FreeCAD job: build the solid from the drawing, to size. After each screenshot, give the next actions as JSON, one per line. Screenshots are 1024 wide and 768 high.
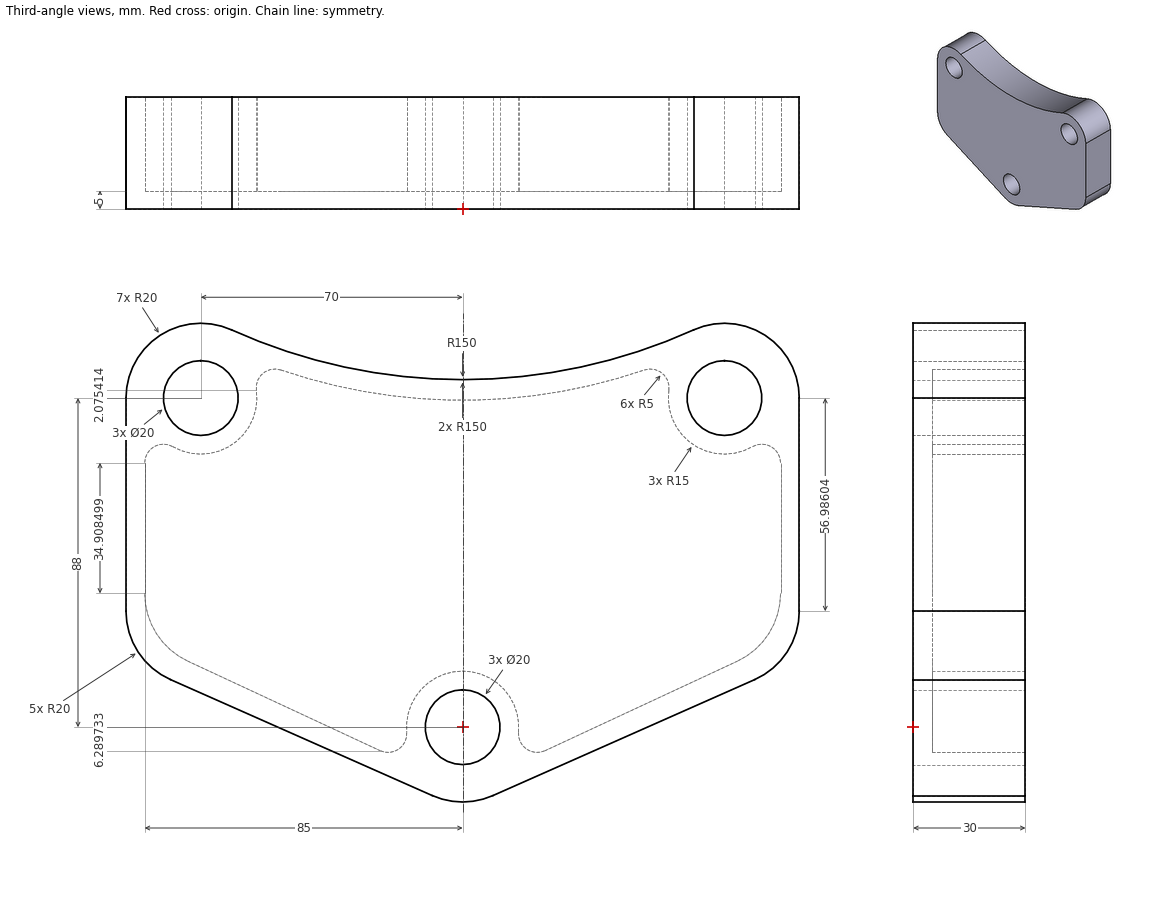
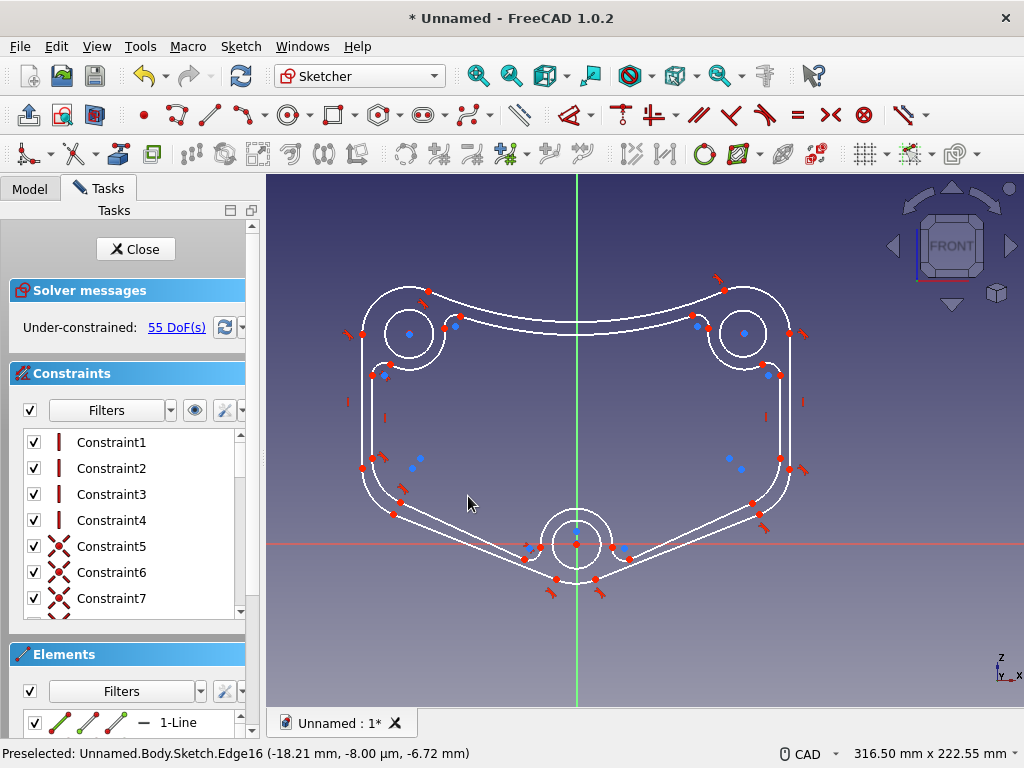
{"action": "scroll", "coordinate": [666, 543], "scroll_direction": "up", "scroll_amount": 3}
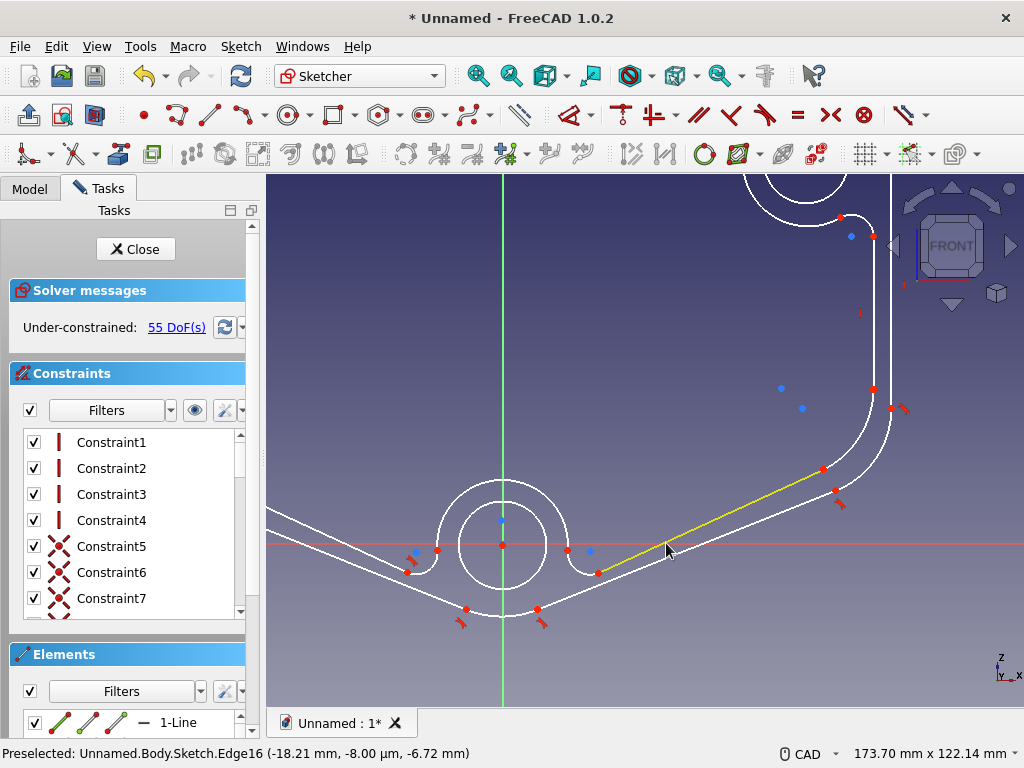
{"action": "left_click", "coordinate": [666, 542]}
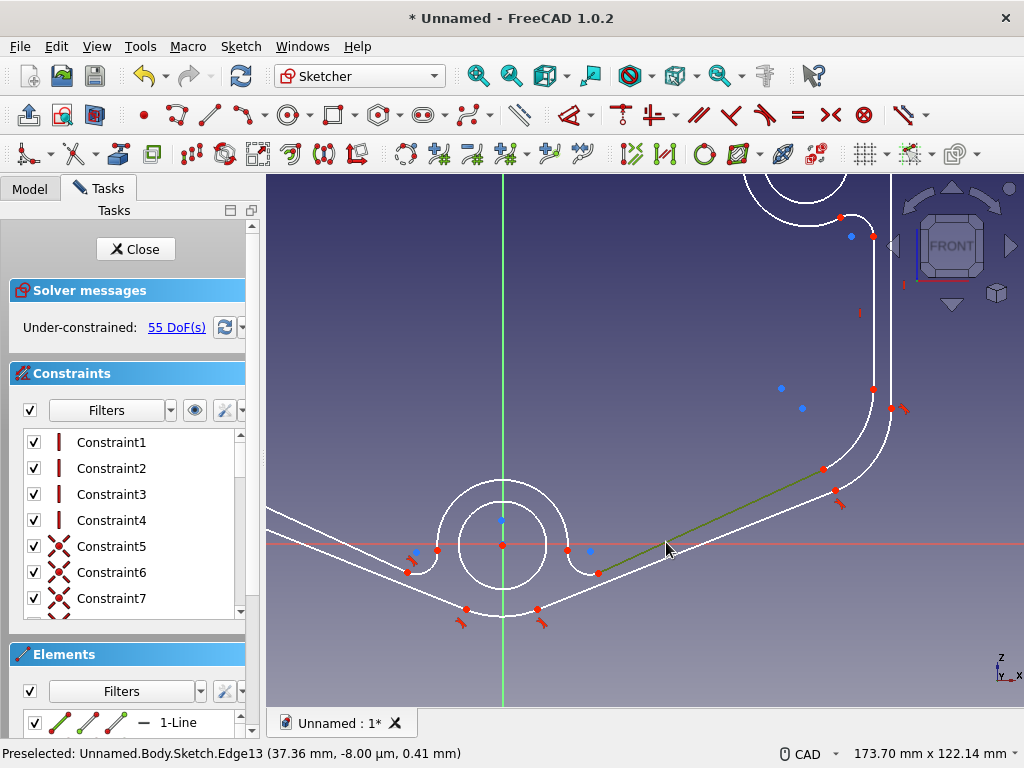
{"action": "left_click", "coordinate": [571, 563]}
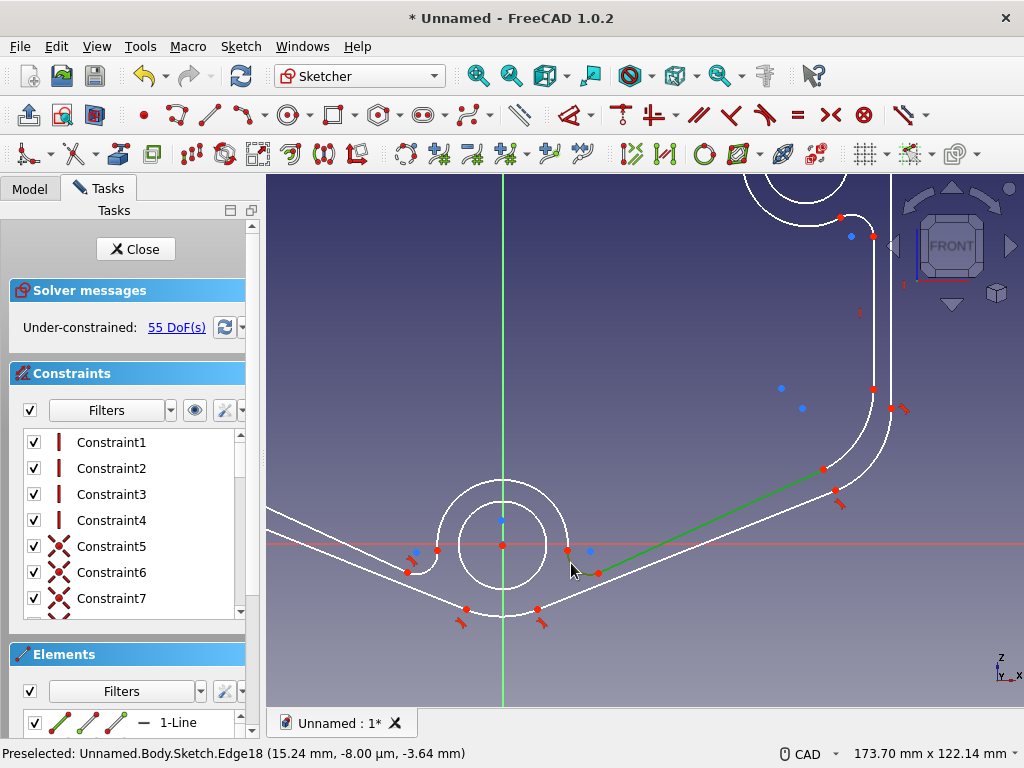
{"action": "left_click", "coordinate": [765, 116]}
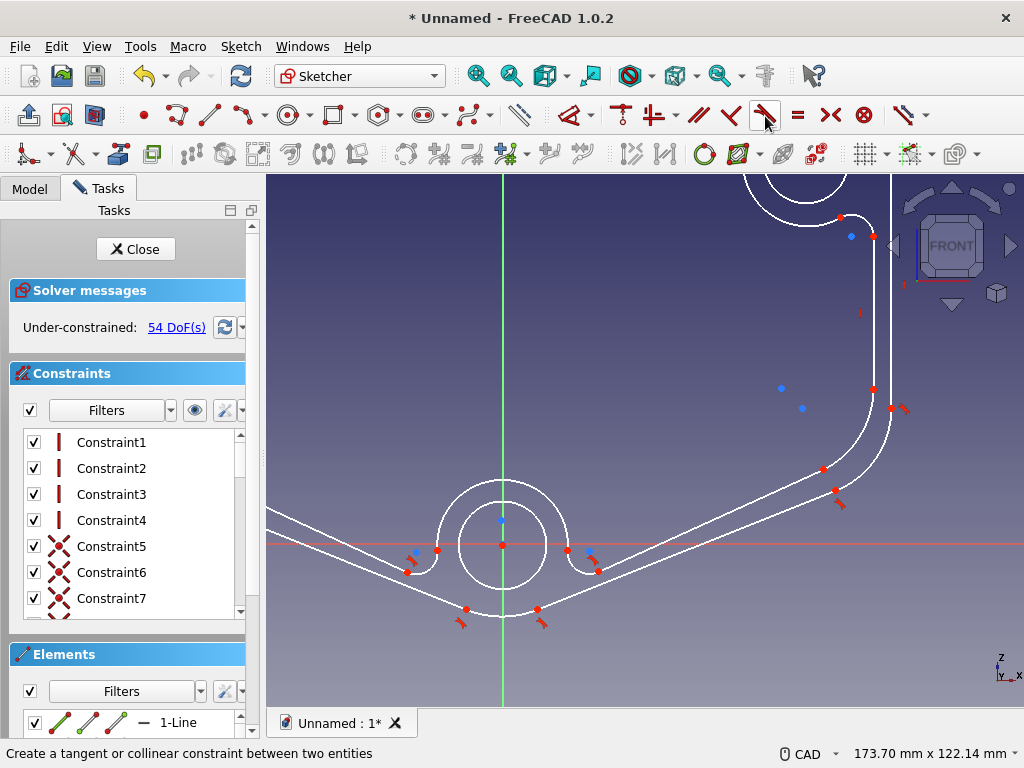
{"action": "left_click", "coordinate": [666, 541]}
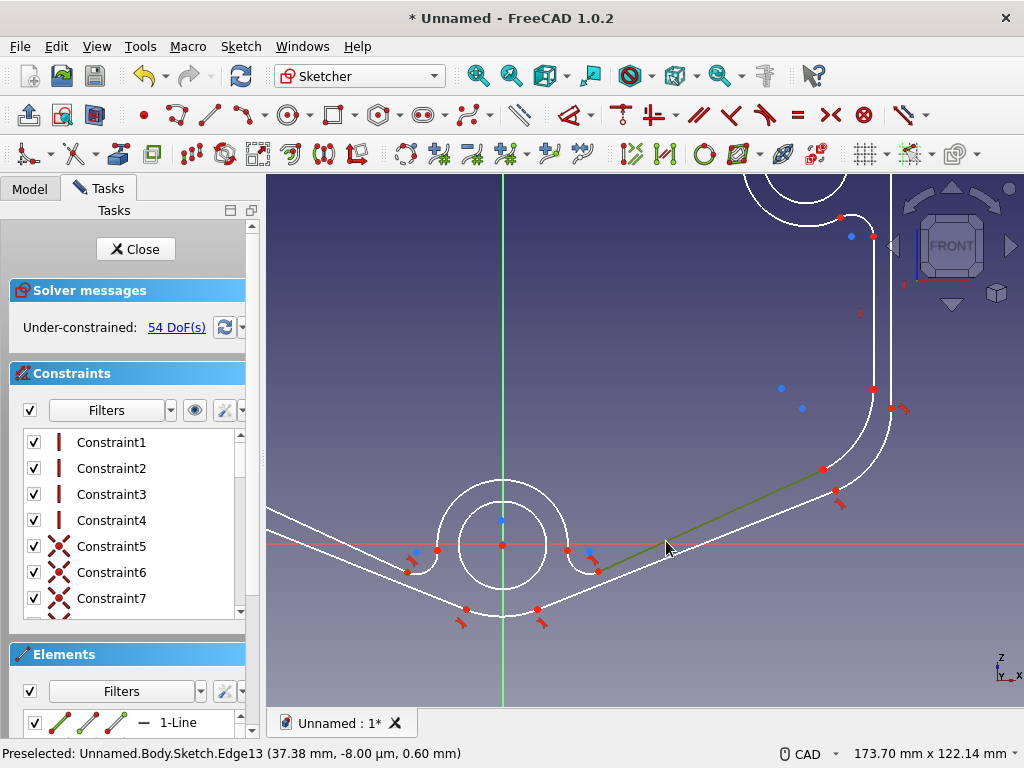
{"action": "left_click", "coordinate": [848, 452]}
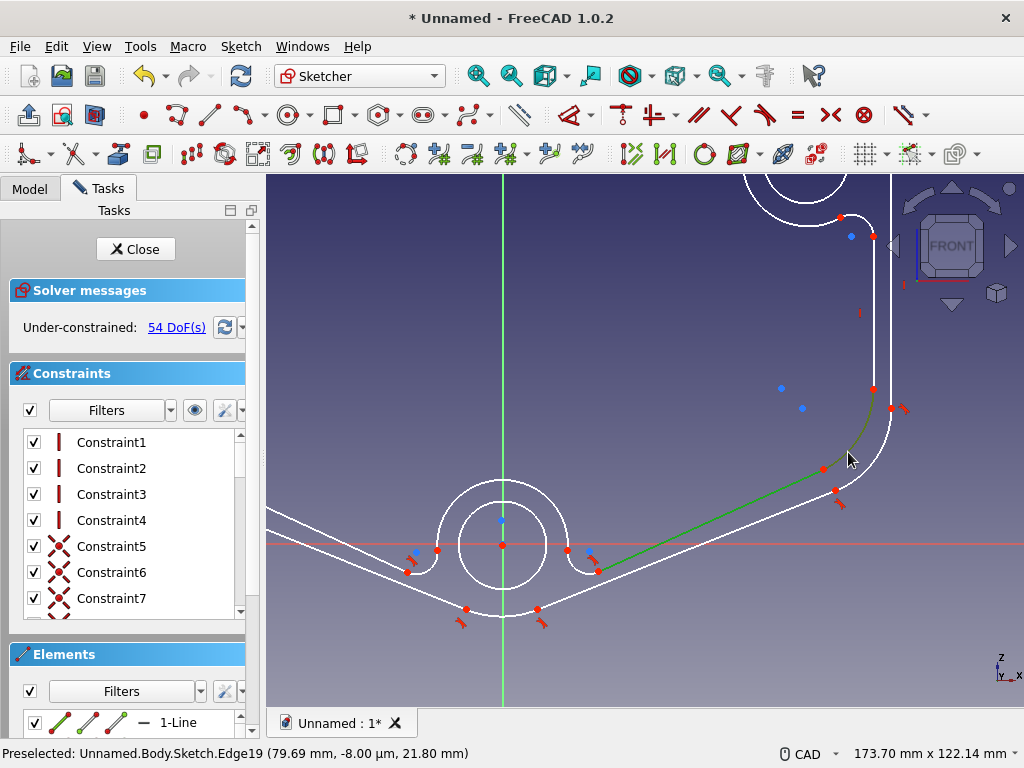
{"action": "left_click", "coordinate": [765, 116]}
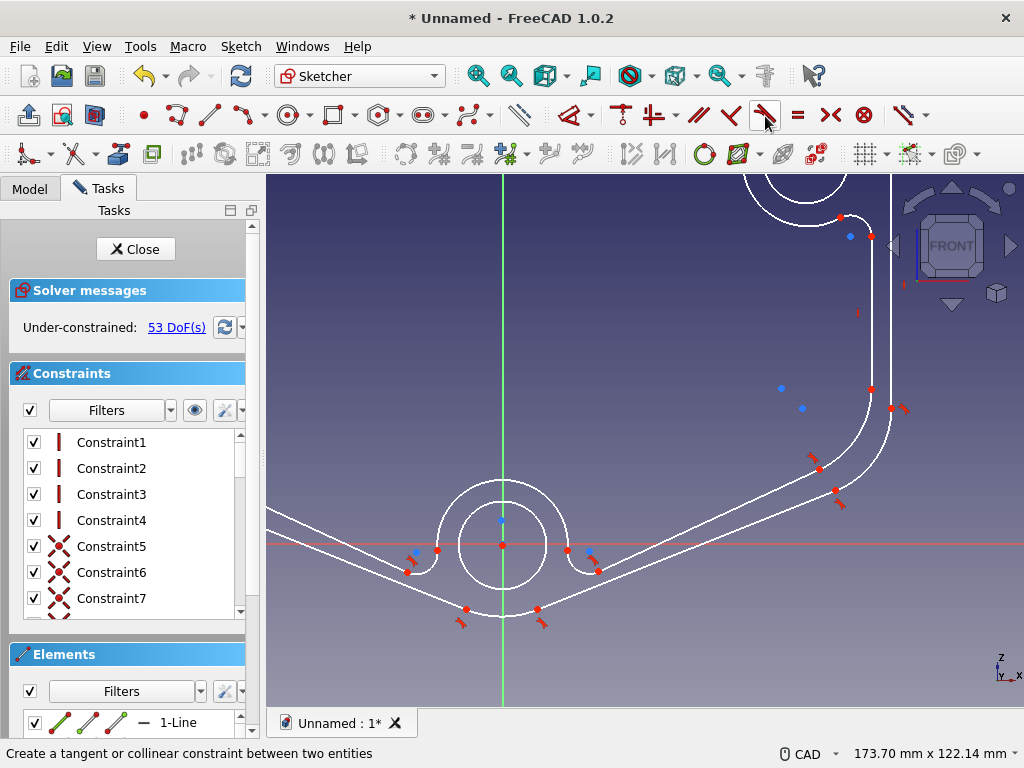
{"action": "scroll", "coordinate": [666, 543], "scroll_direction": "down", "scroll_amount": 3}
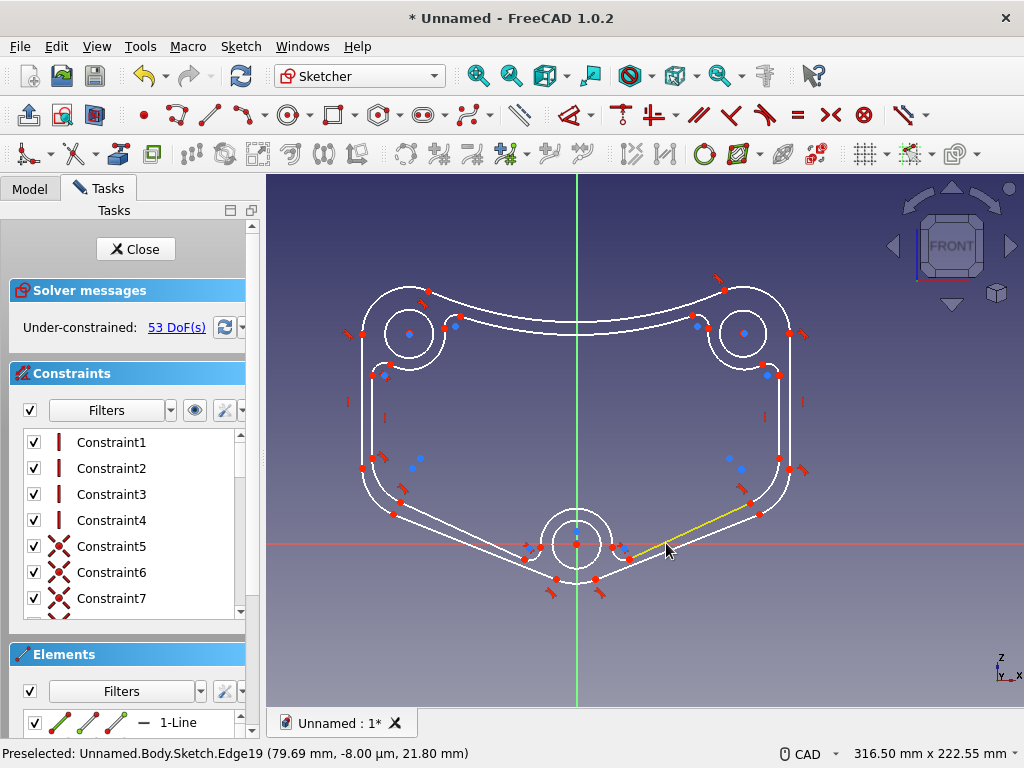
{"action": "scroll", "coordinate": [779, 434], "scroll_direction": "up", "scroll_amount": 2}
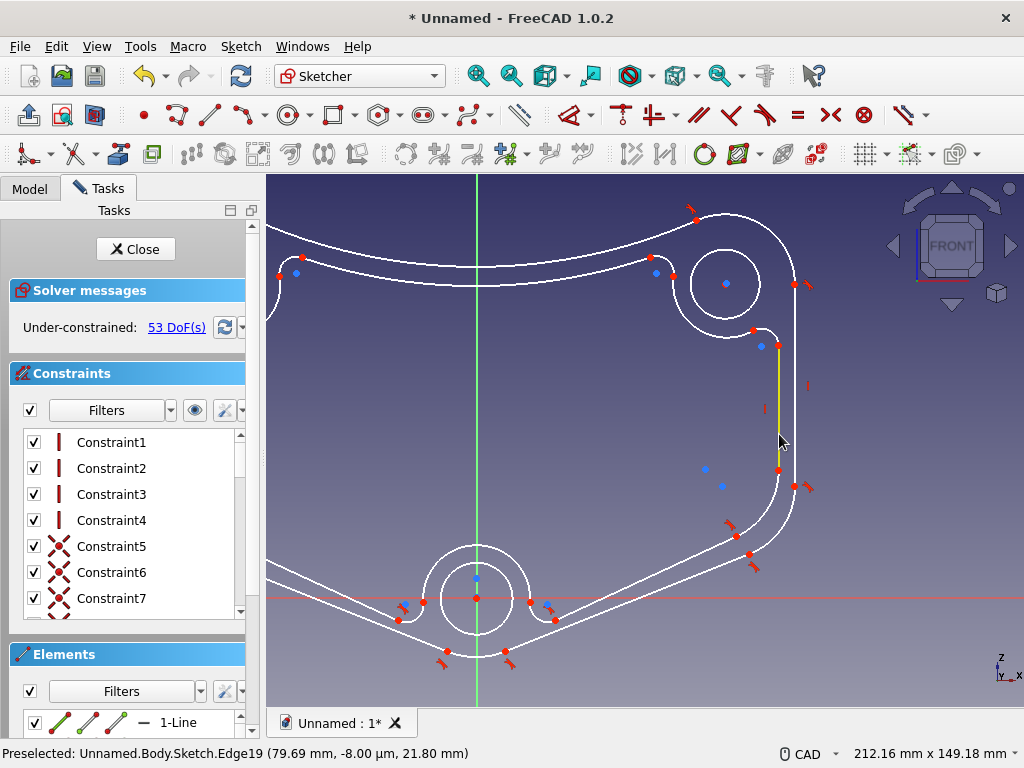
{"action": "left_click", "coordinate": [779, 433]}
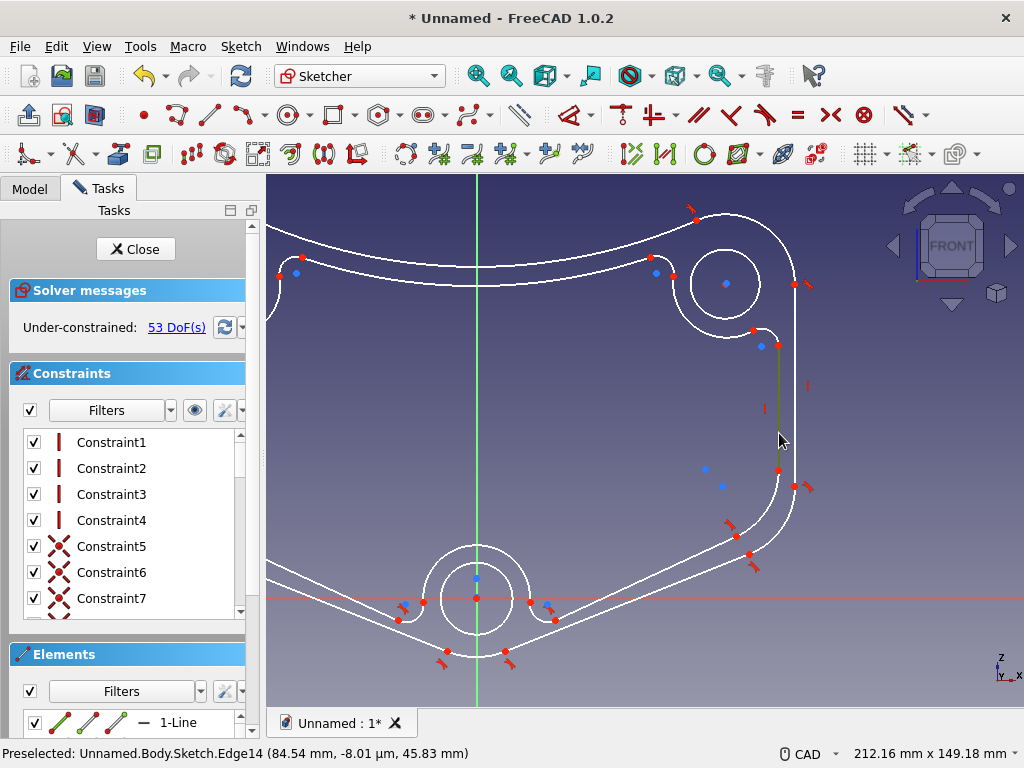
{"action": "left_click", "coordinate": [756, 523]}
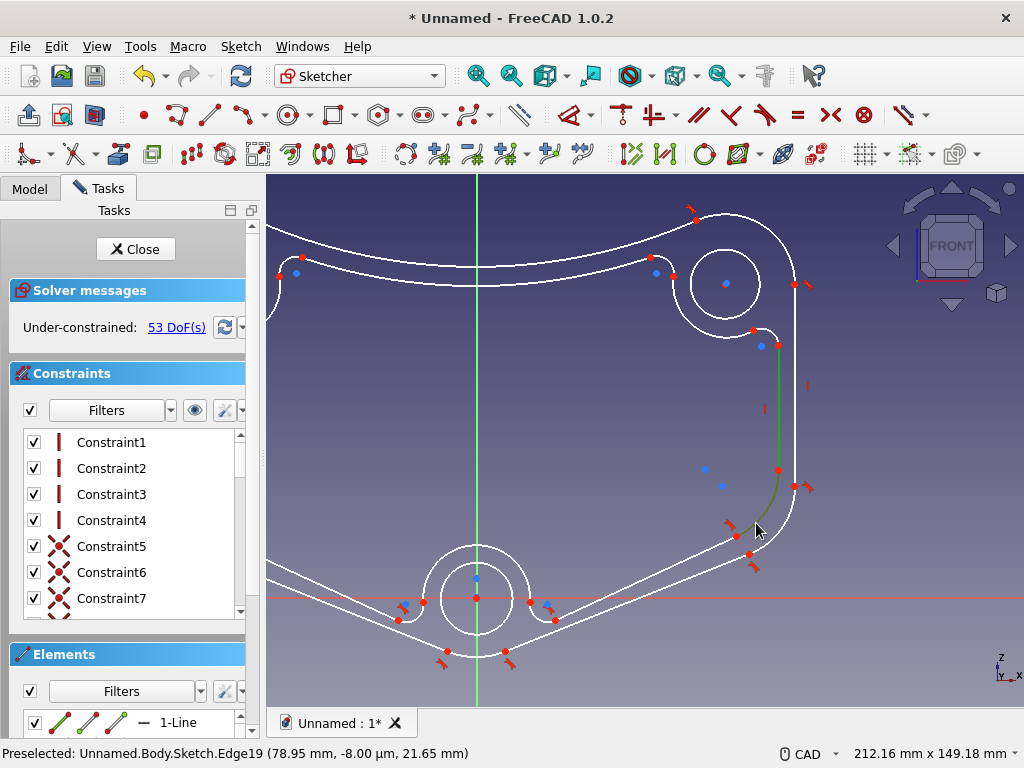
{"action": "left_click", "coordinate": [765, 116]}